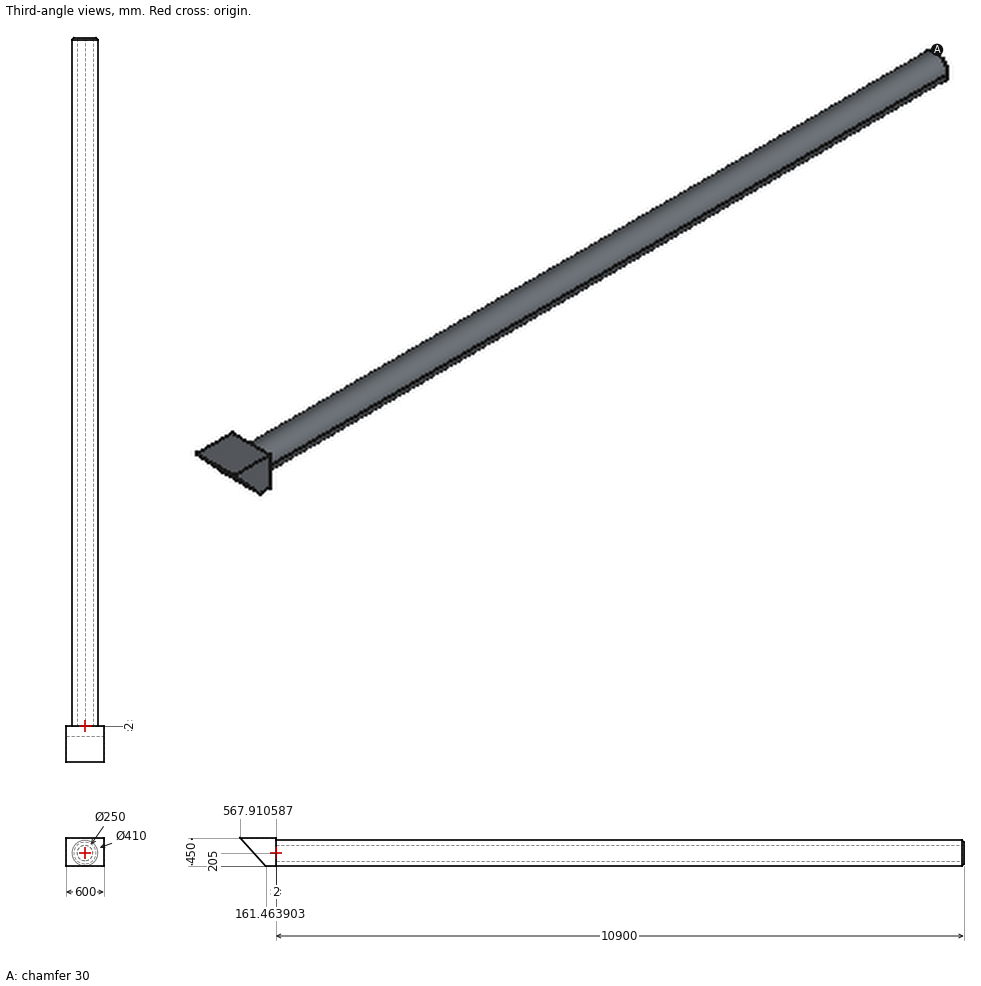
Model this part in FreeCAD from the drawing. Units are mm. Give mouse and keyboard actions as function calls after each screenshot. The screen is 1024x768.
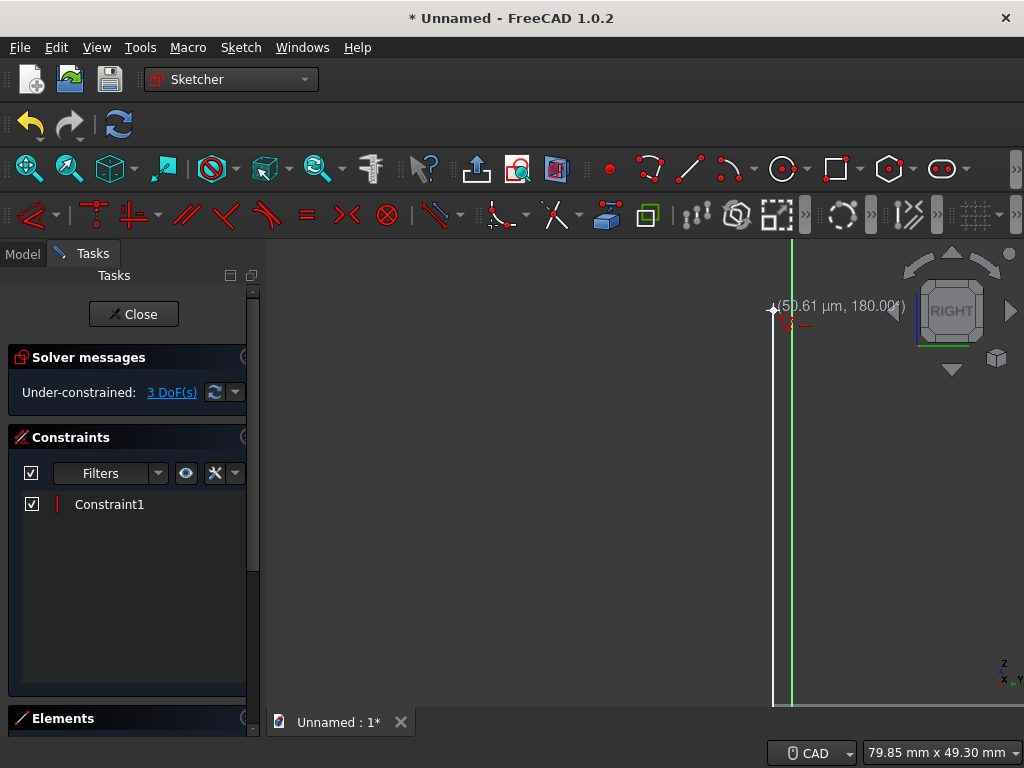
scroll(776, 315, down, 13)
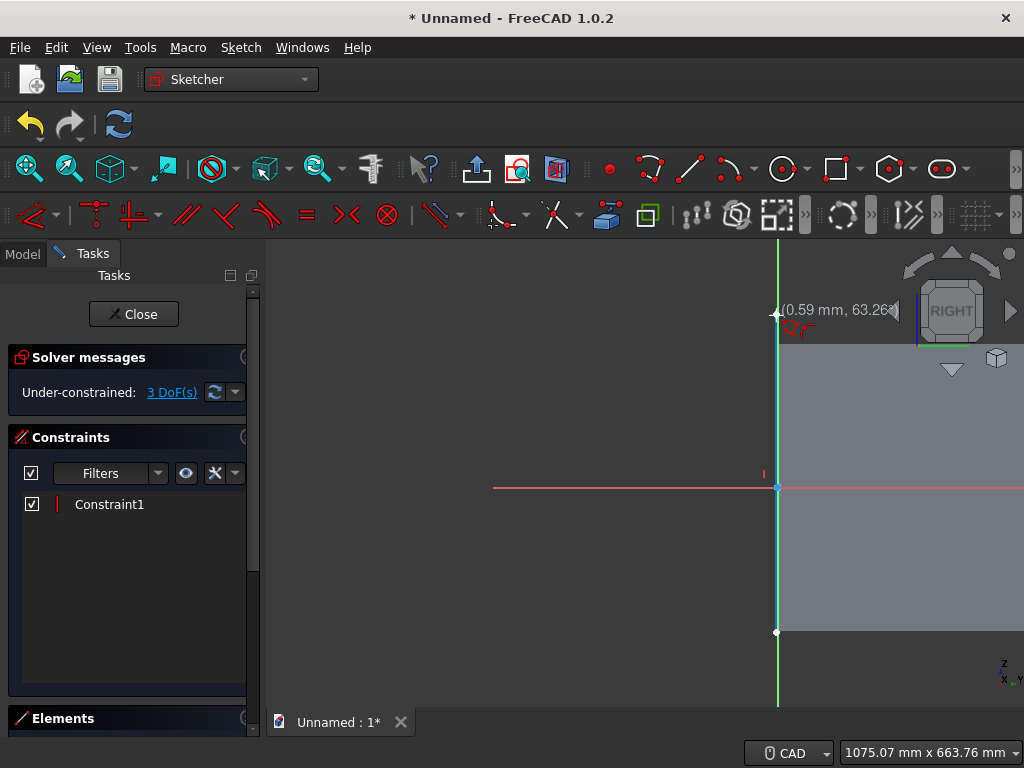
click(376, 315)
click(663, 632)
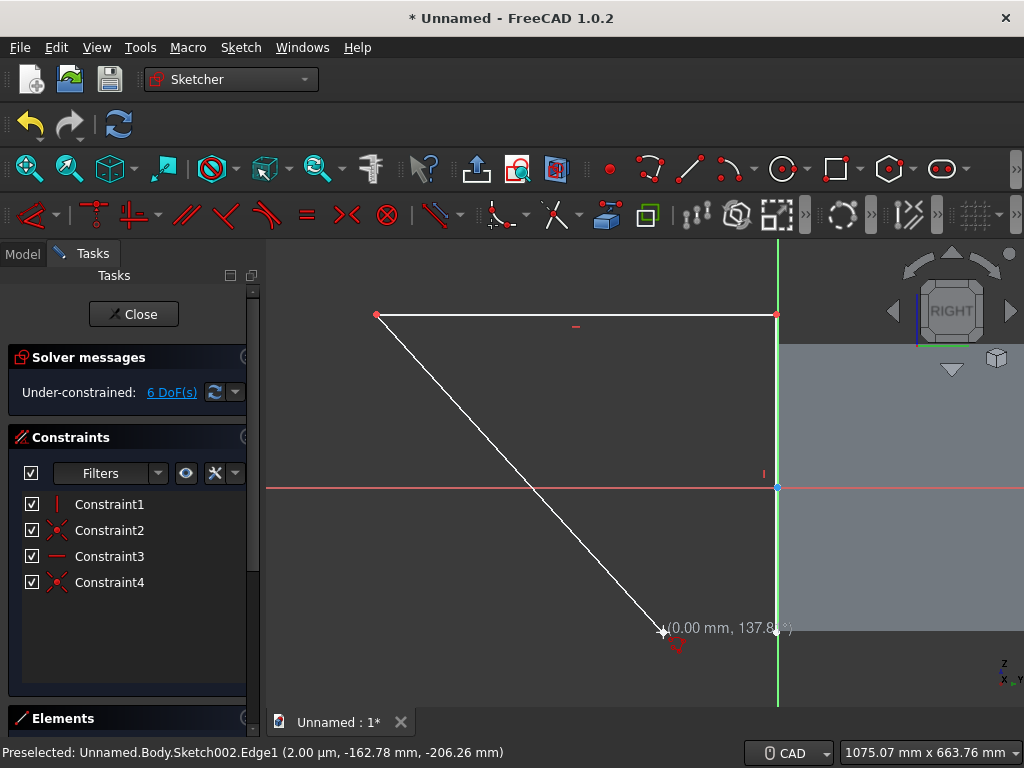
scroll(776, 632, up, 13)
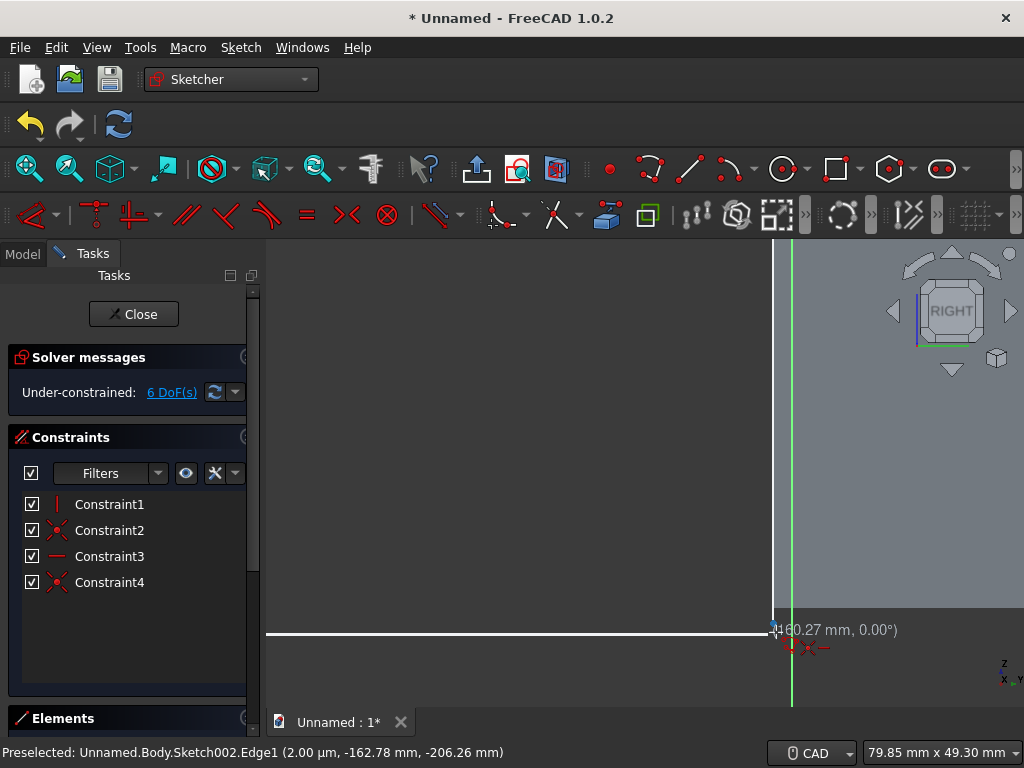
click(773, 623)
key(Escape)
key(Escape)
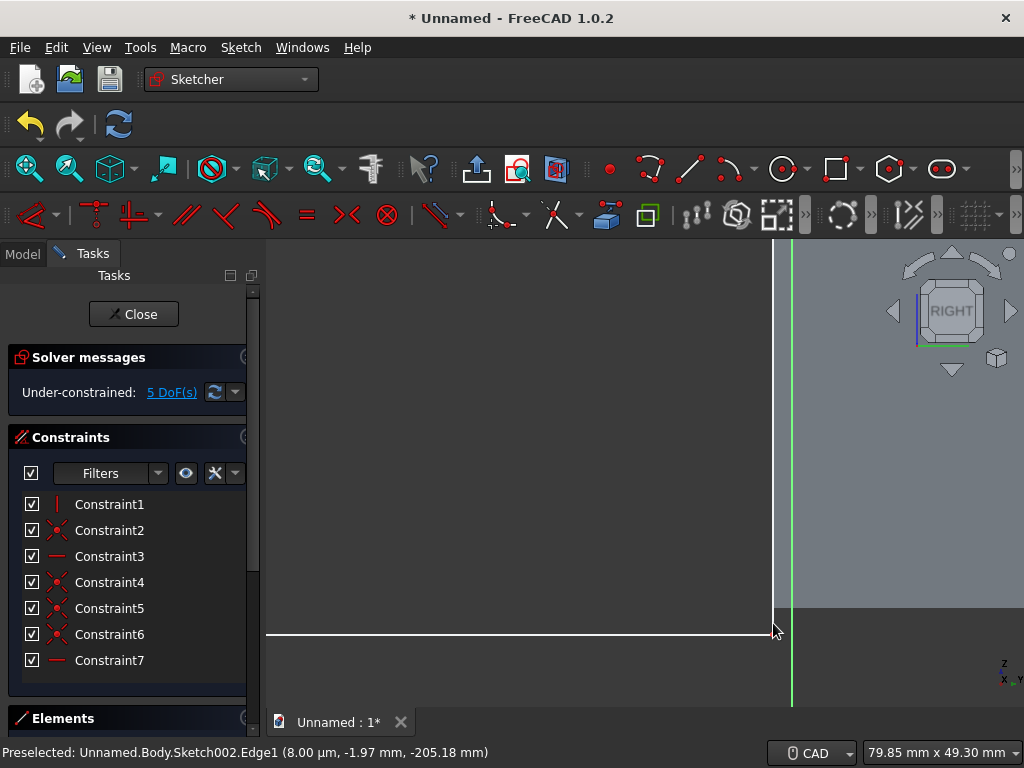
click(32, 216)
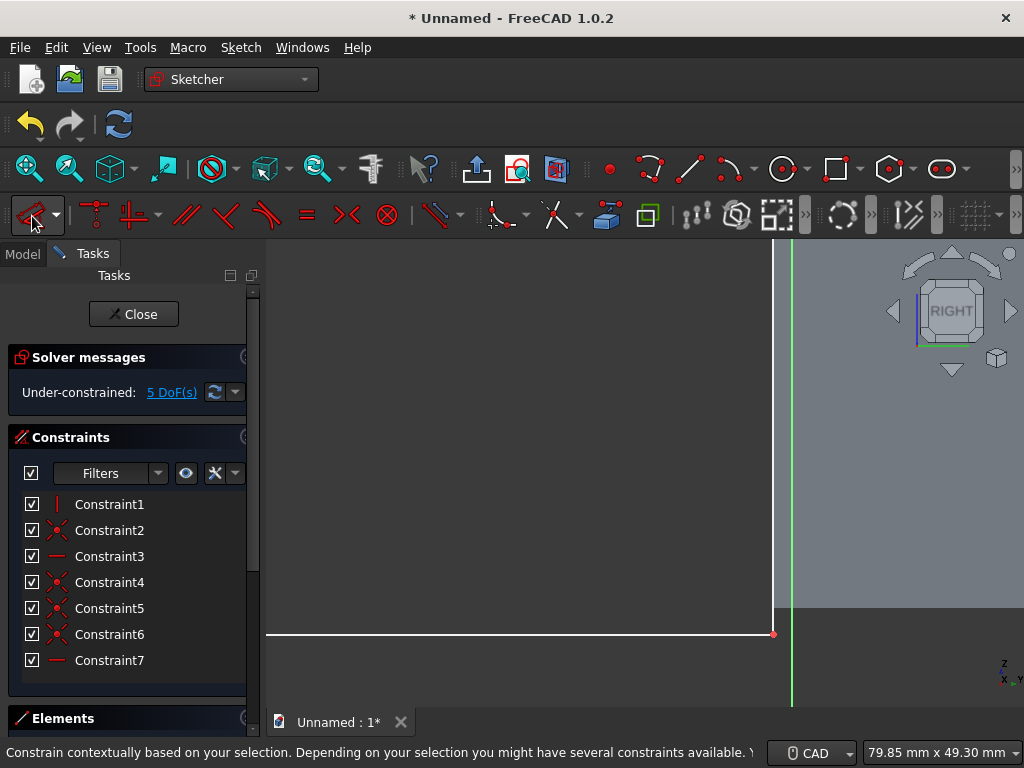
scroll(773, 635, up, 4)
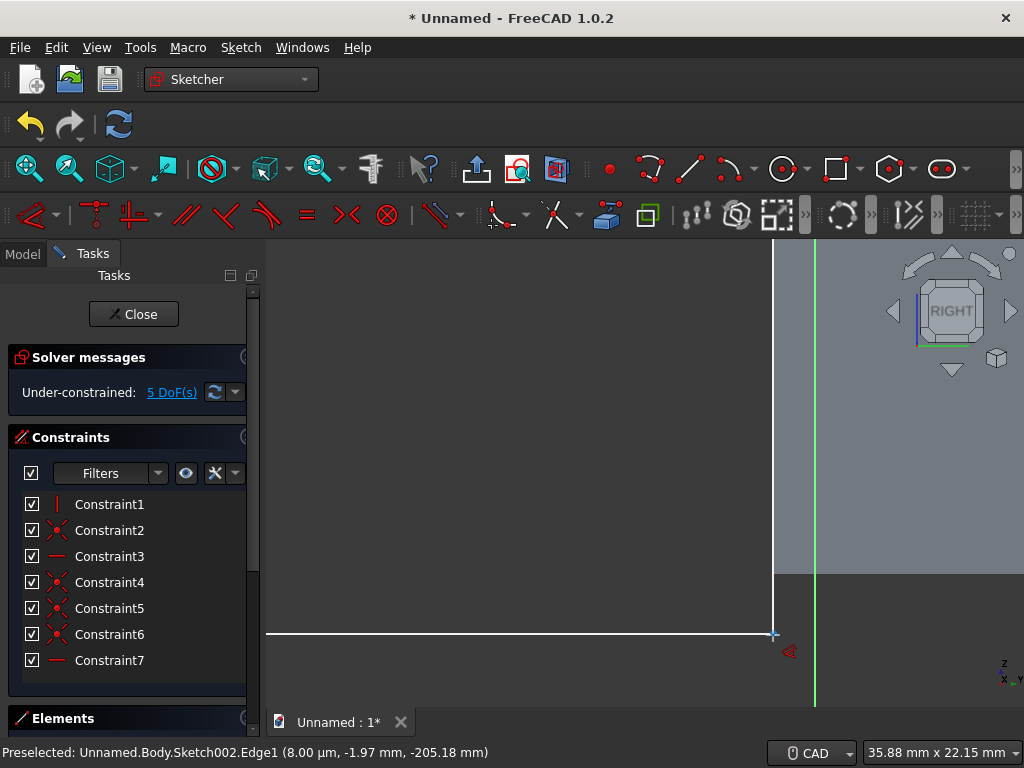
click(773, 634)
click(794, 668)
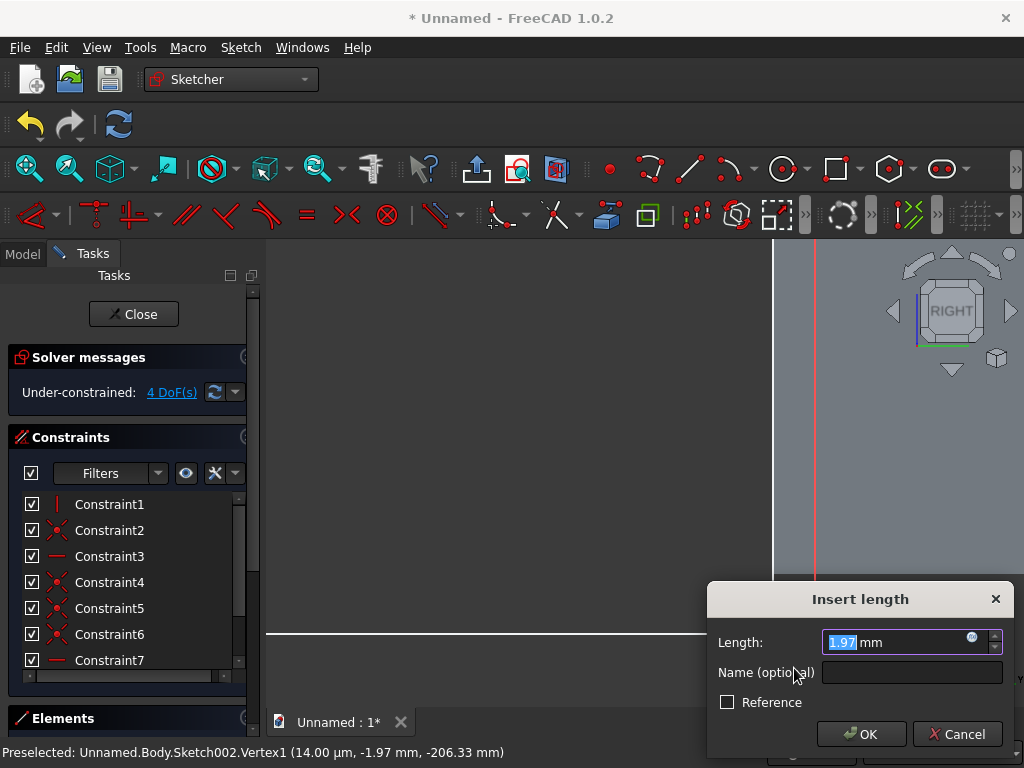
text(2)
key(Return)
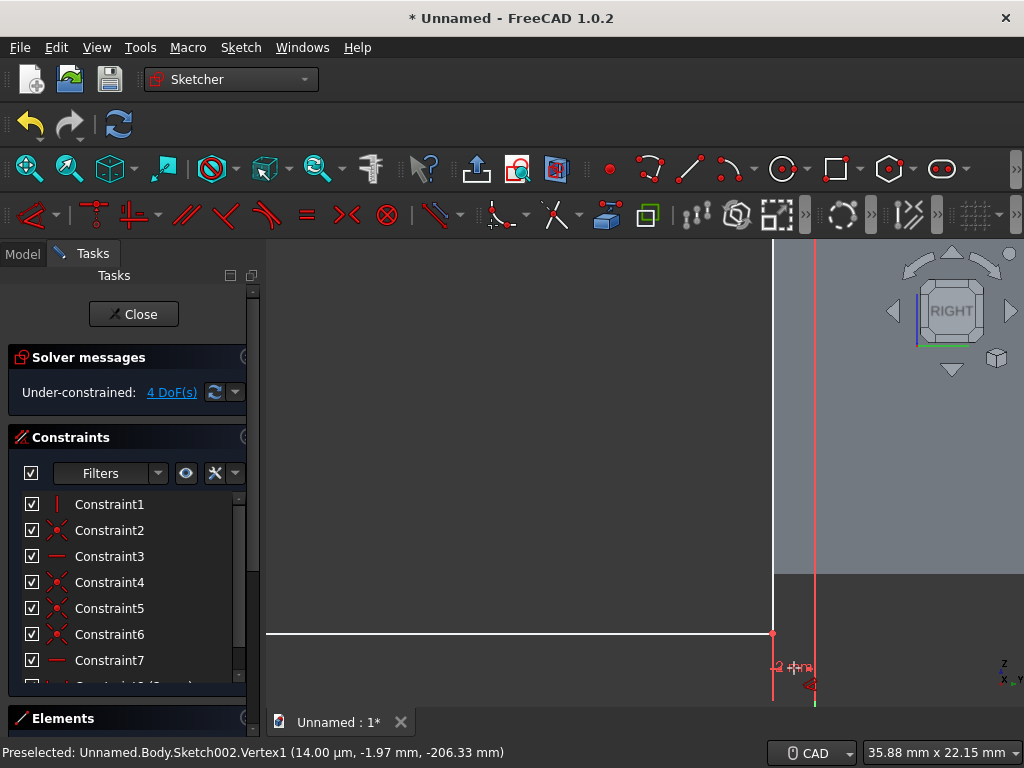
scroll(776, 633, down, 17)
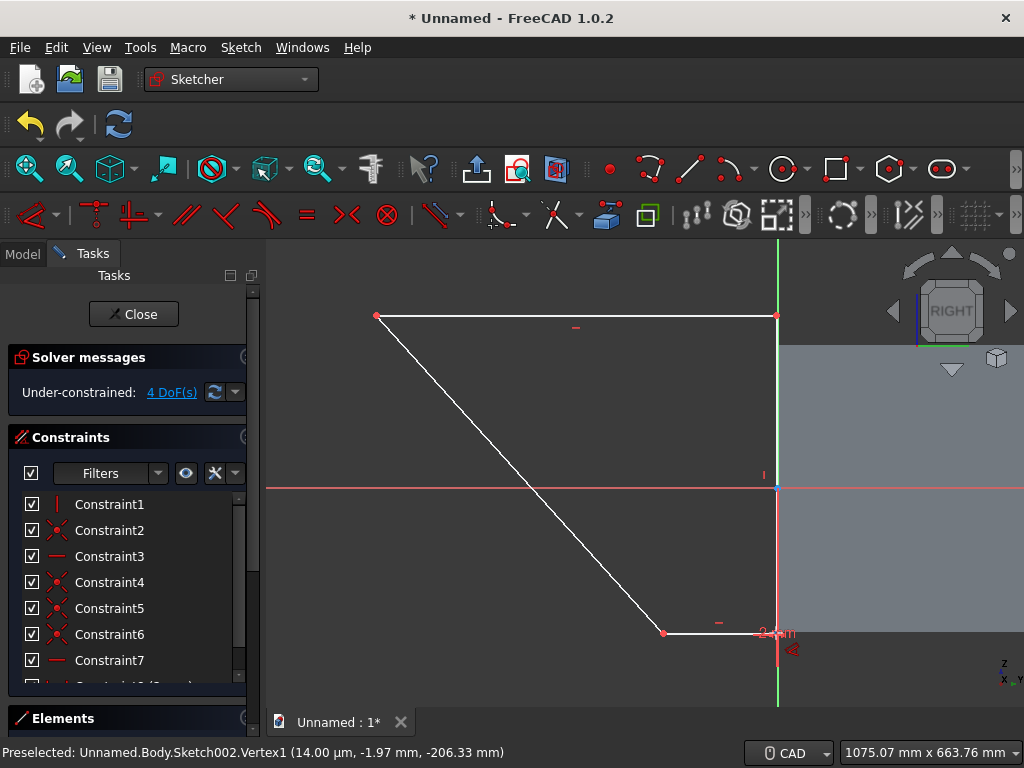
scroll(777, 538, up, 12)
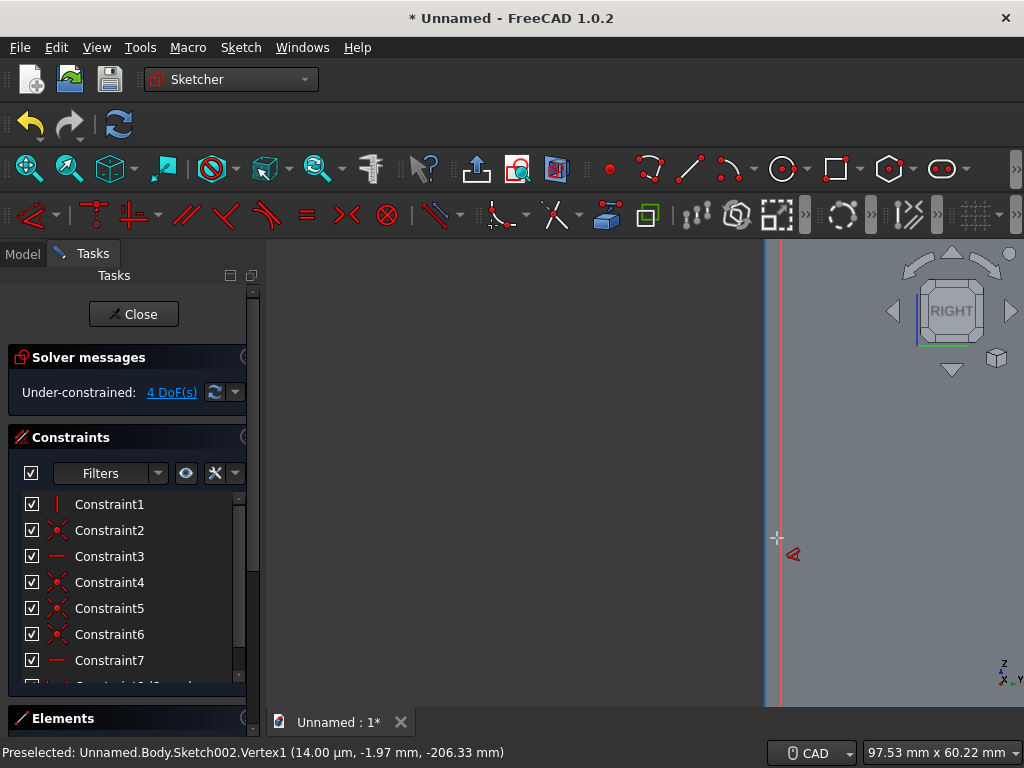
click(765, 536)
click(799, 473)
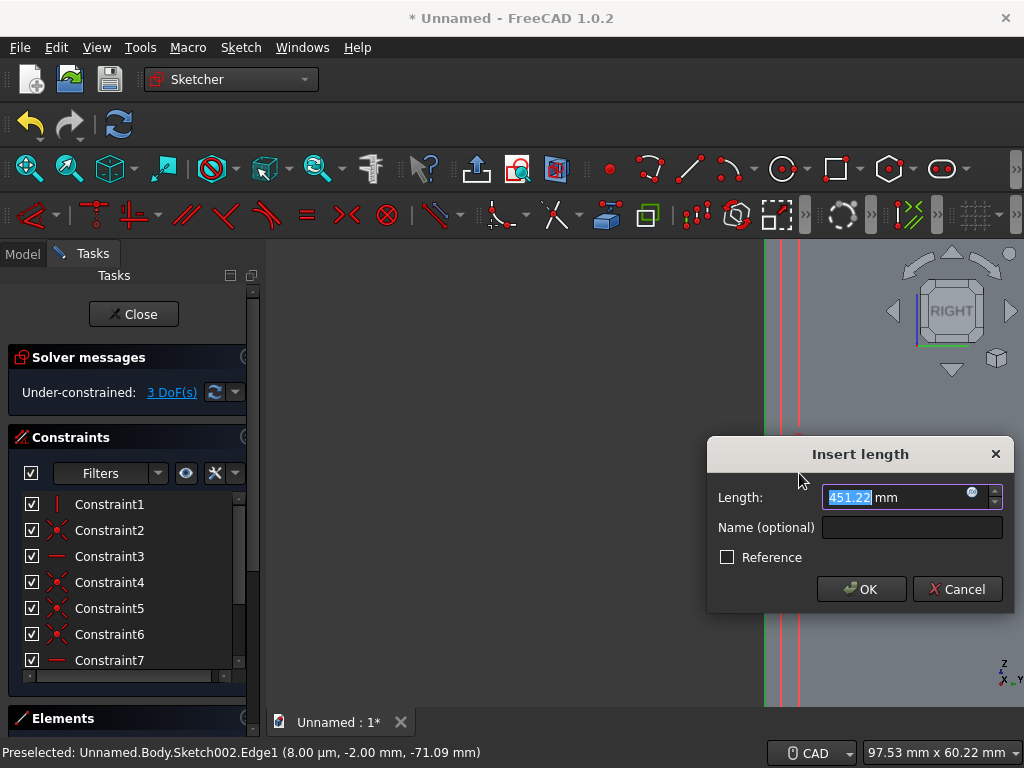
text(450)
key(Return)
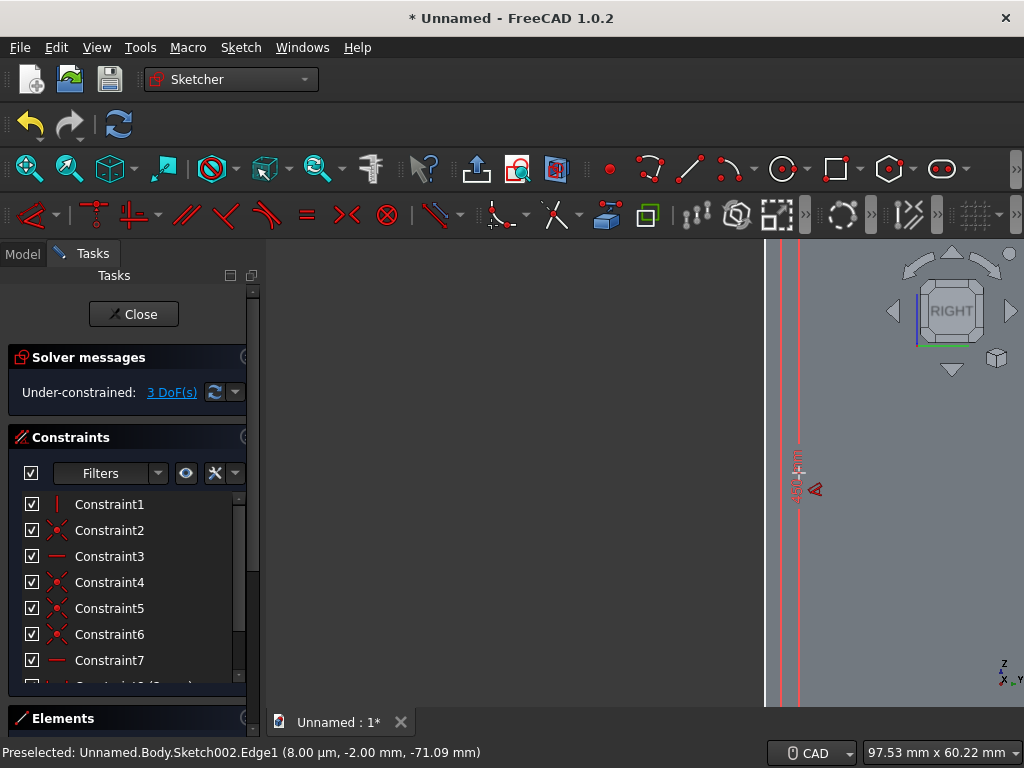
scroll(777, 537, down, 12)